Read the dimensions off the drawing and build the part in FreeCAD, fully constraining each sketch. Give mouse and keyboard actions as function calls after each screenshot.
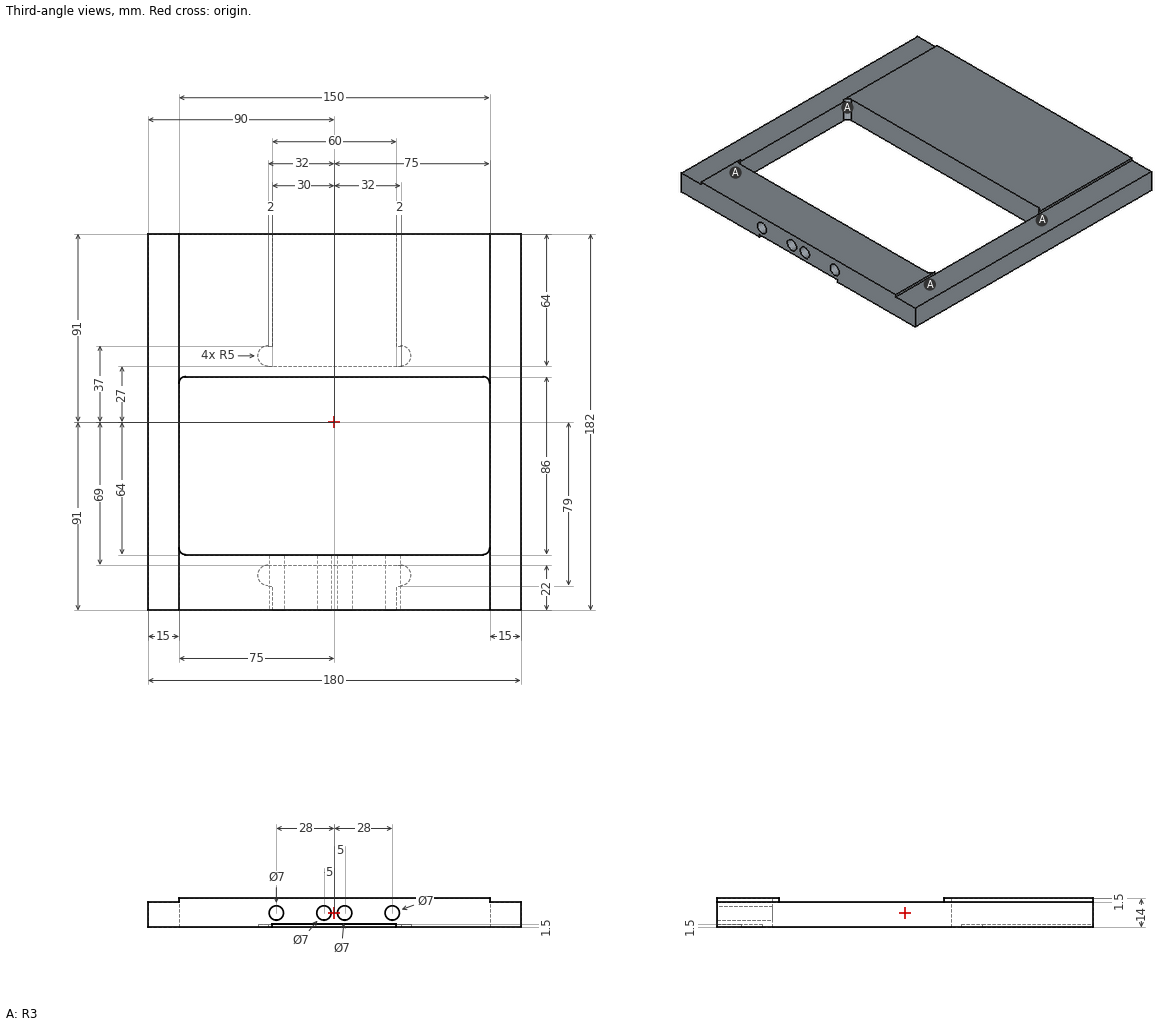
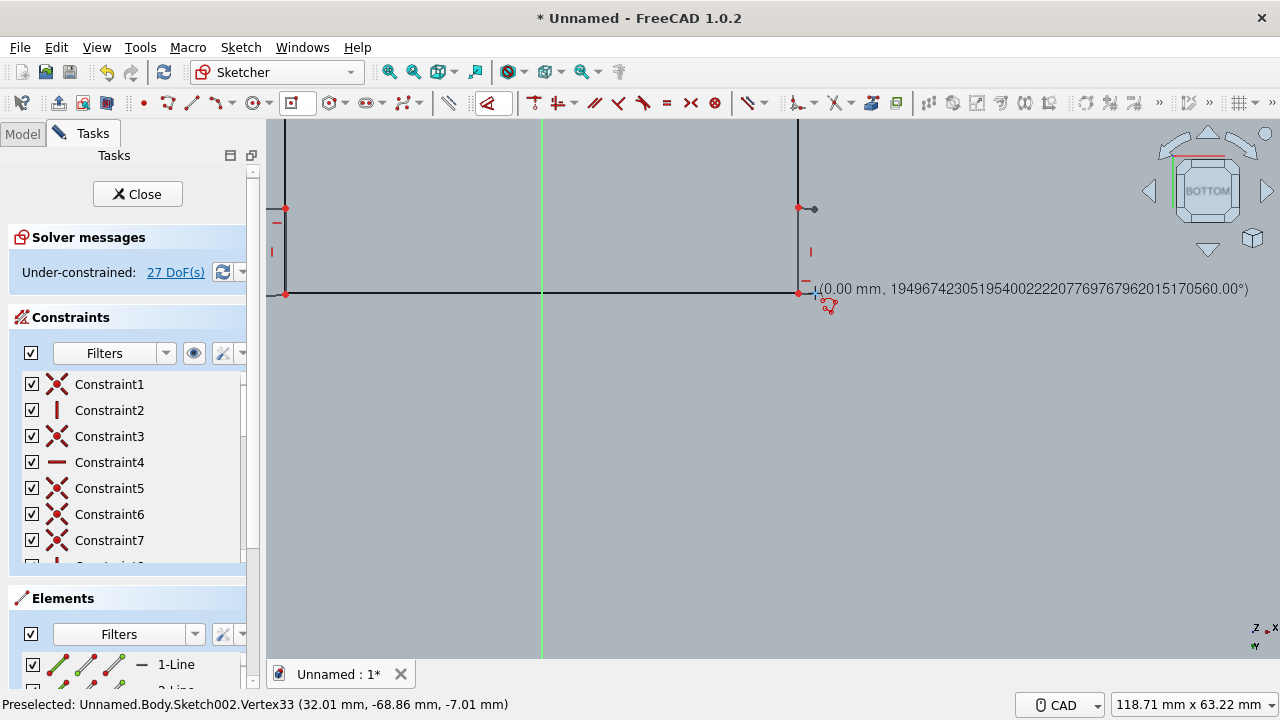
key(g)
key(3)
key(a)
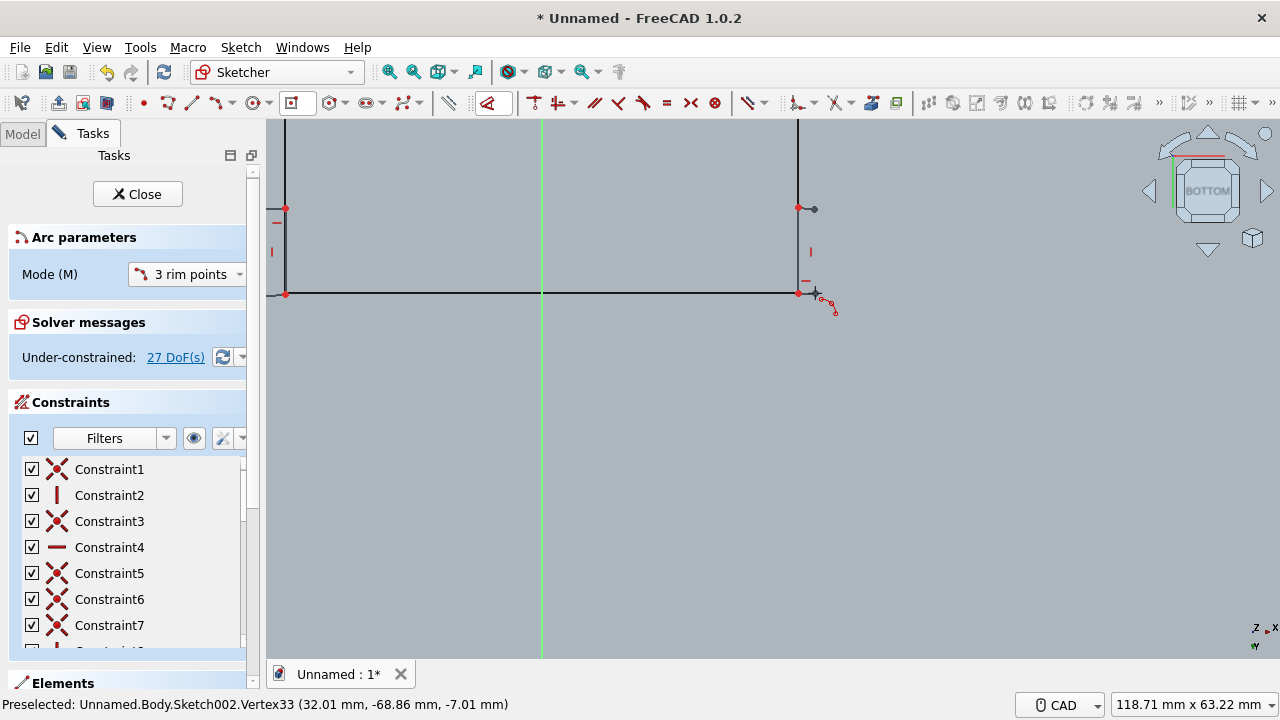
scroll(815, 293, up, 4)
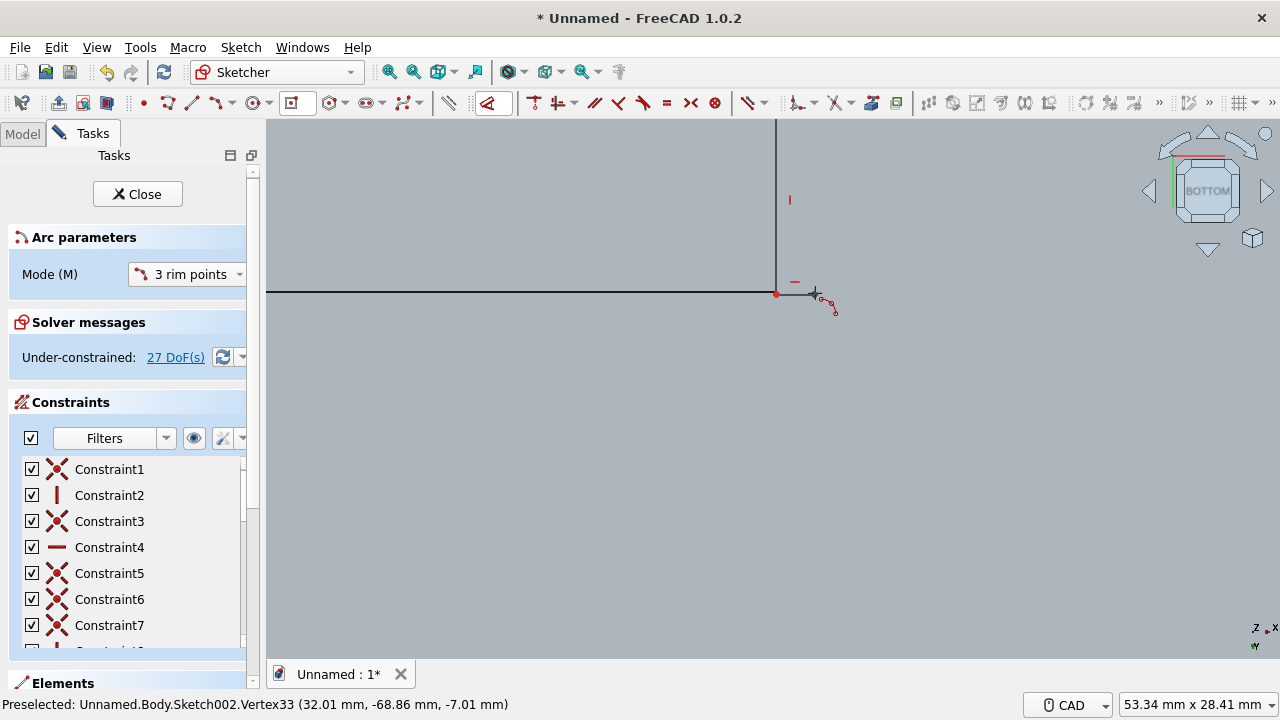
click(814, 295)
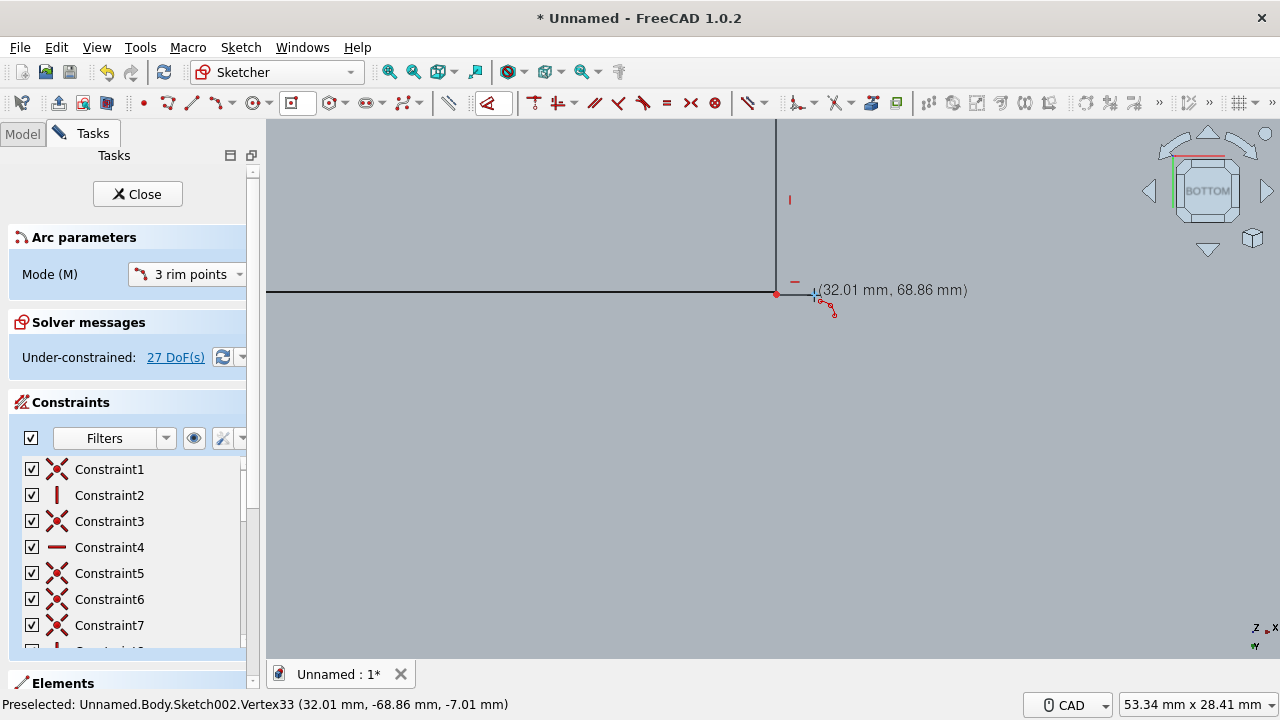
scroll(803, 227, down, 9)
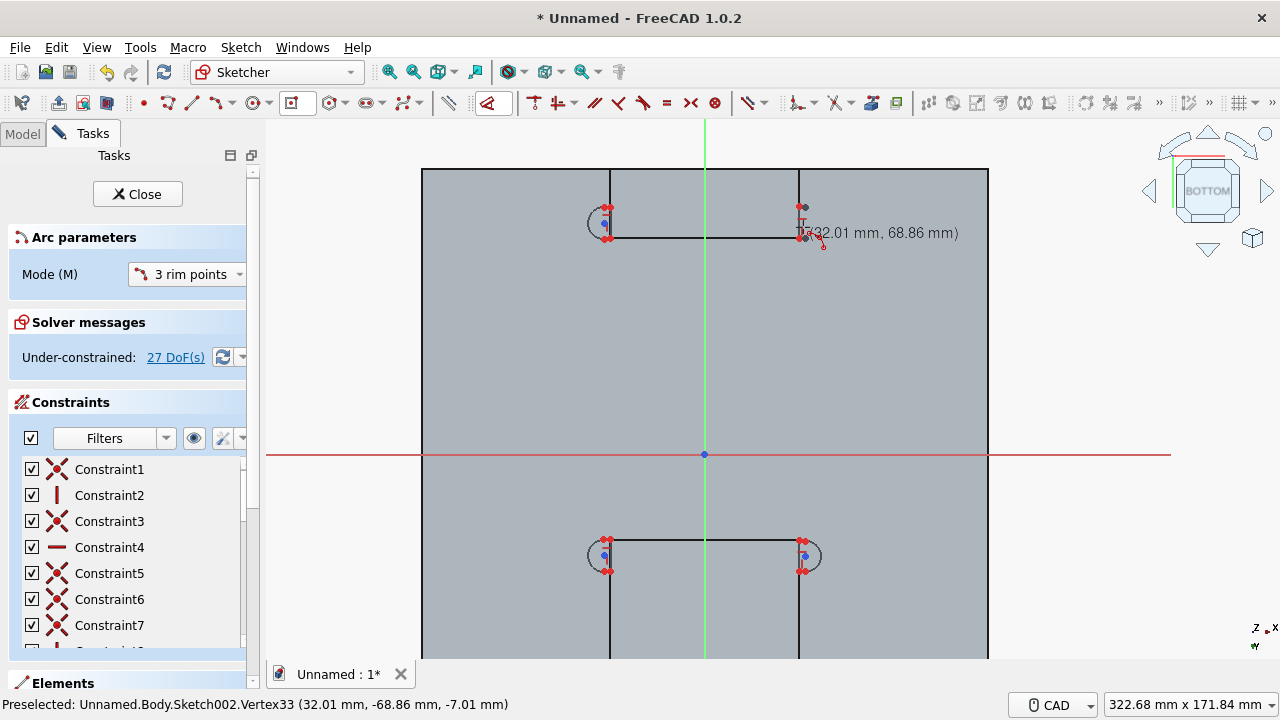
scroll(805, 207, up, 9)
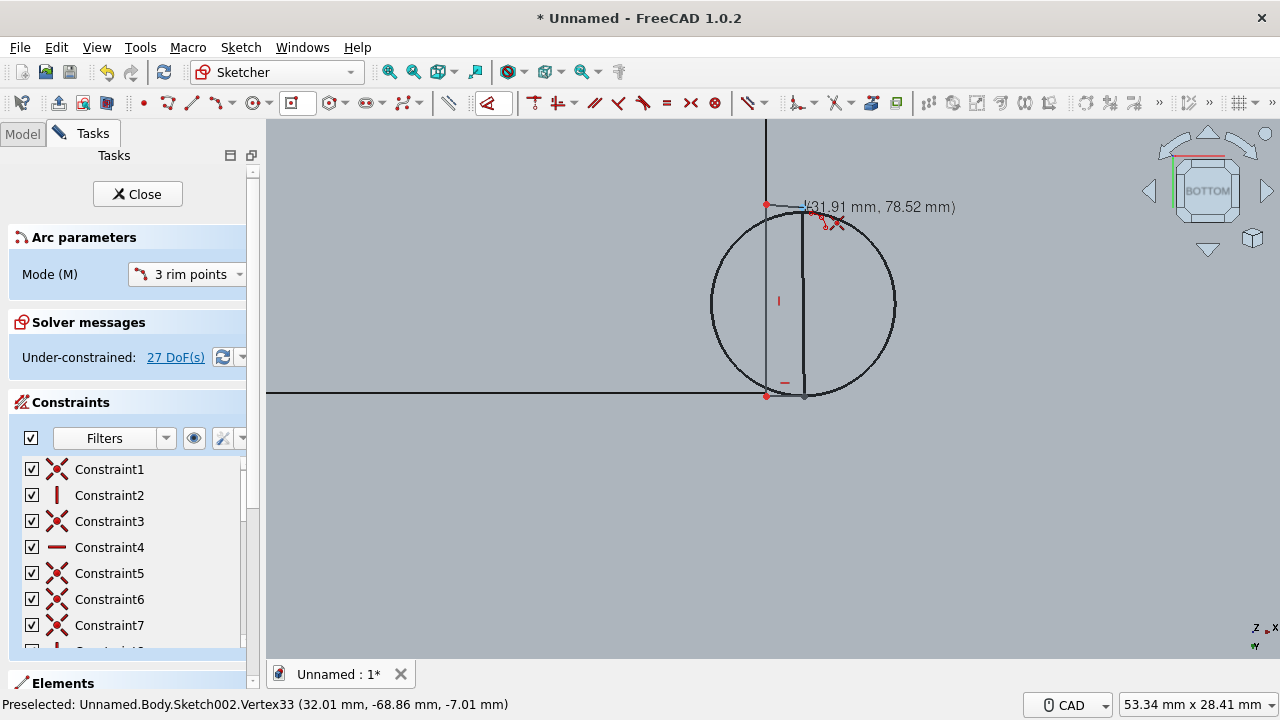
click(803, 208)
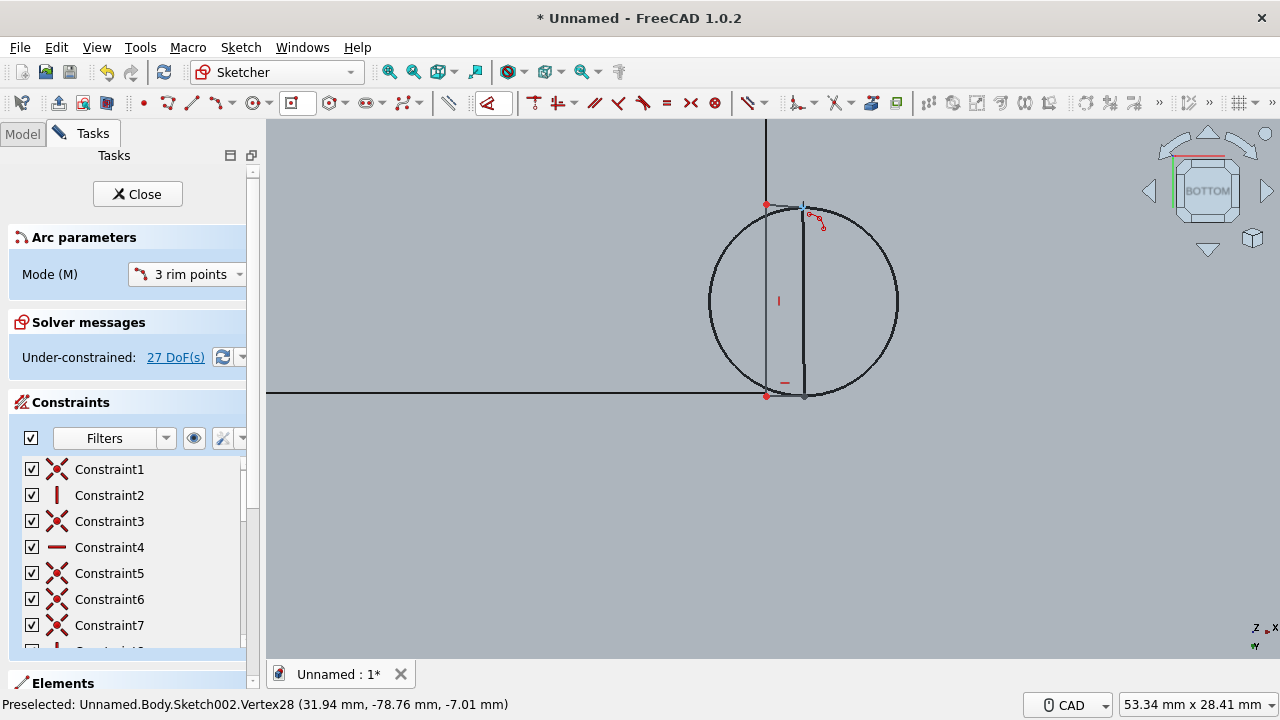
scroll(805, 207, down, 9)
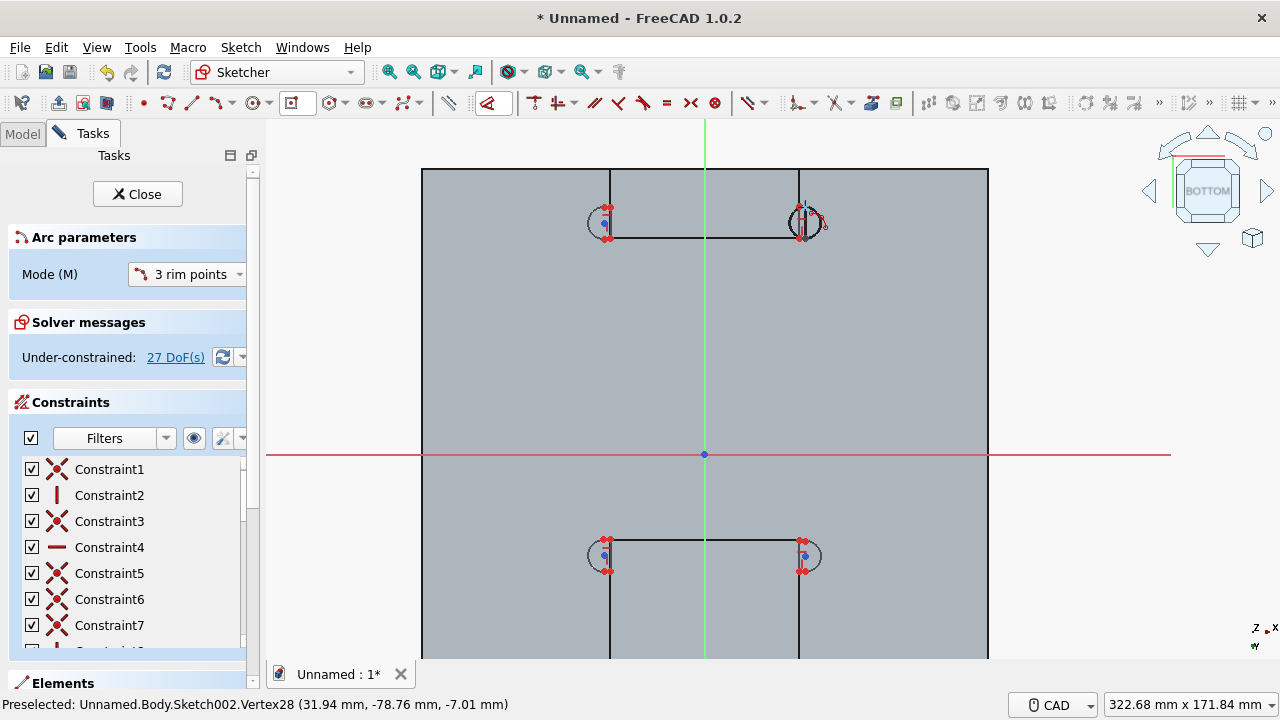
click(821, 222)
key(Escape)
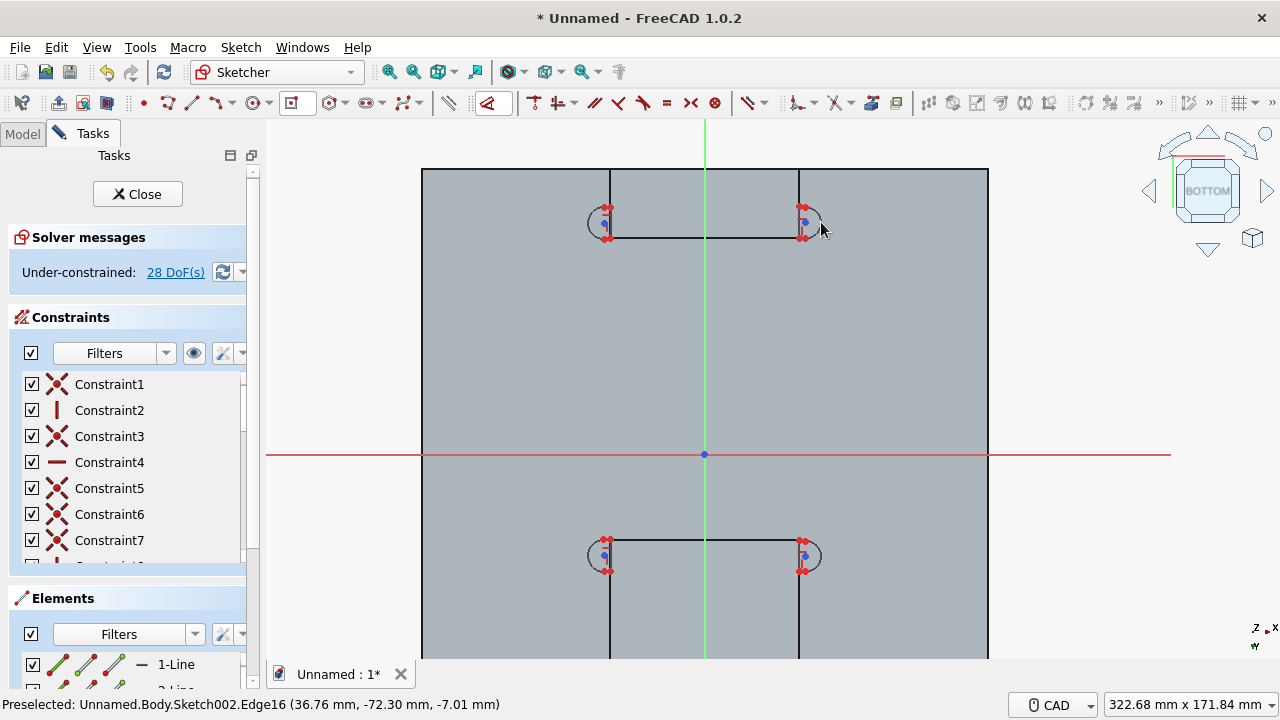
scroll(608, 572, up, 8)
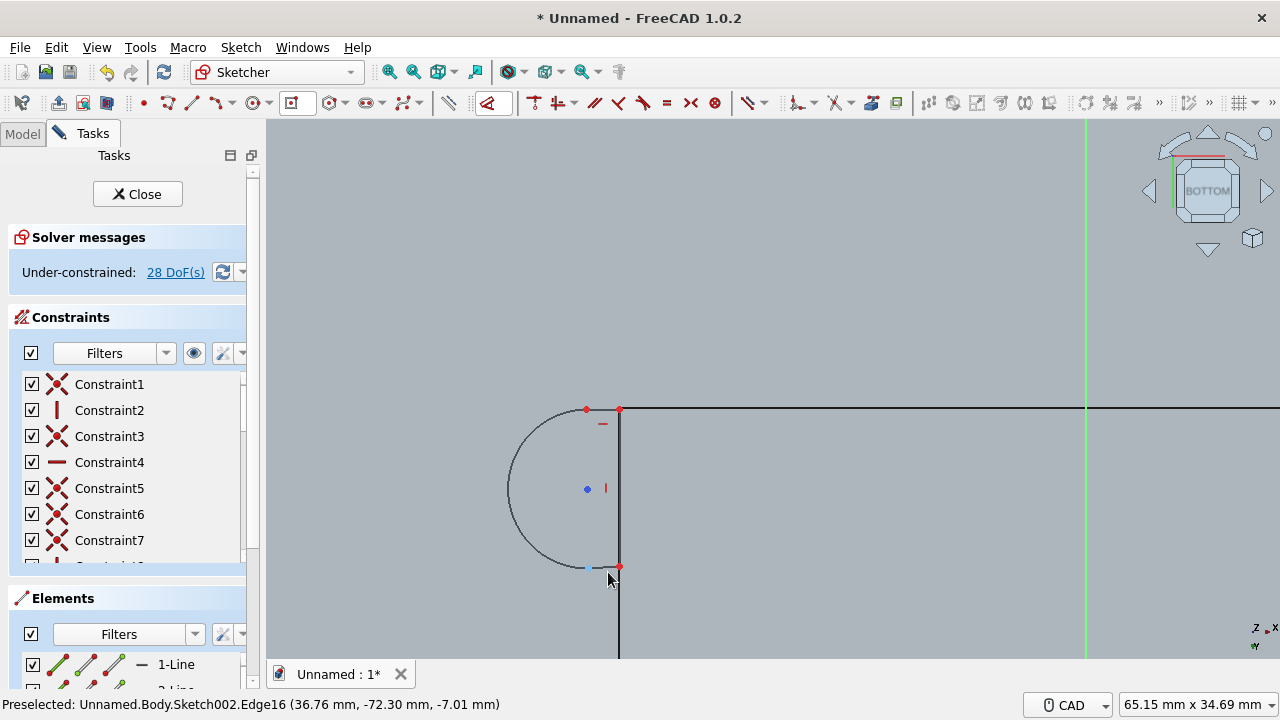
click(604, 567)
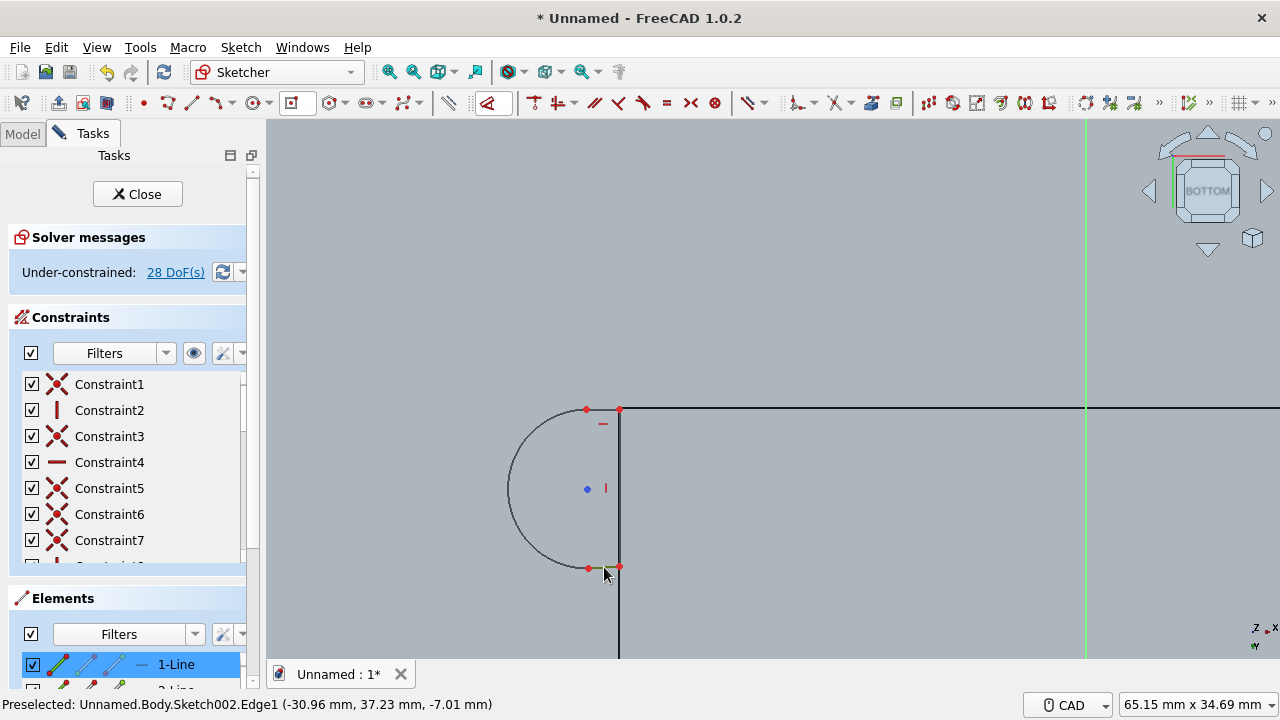
scroll(608, 573, down, 8)